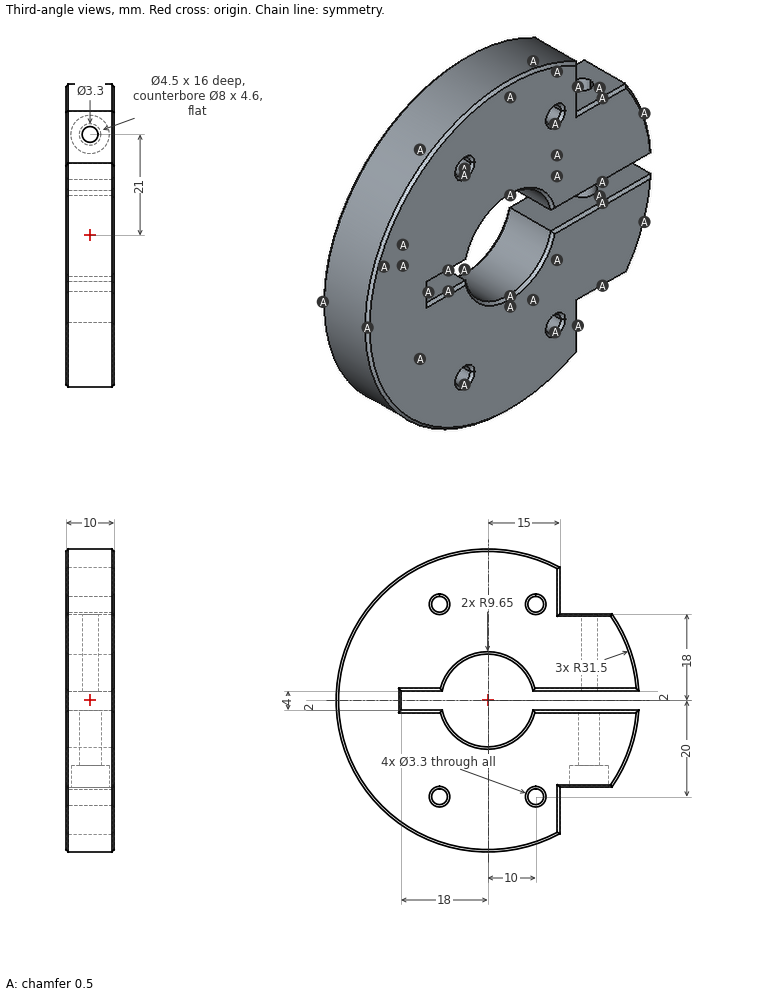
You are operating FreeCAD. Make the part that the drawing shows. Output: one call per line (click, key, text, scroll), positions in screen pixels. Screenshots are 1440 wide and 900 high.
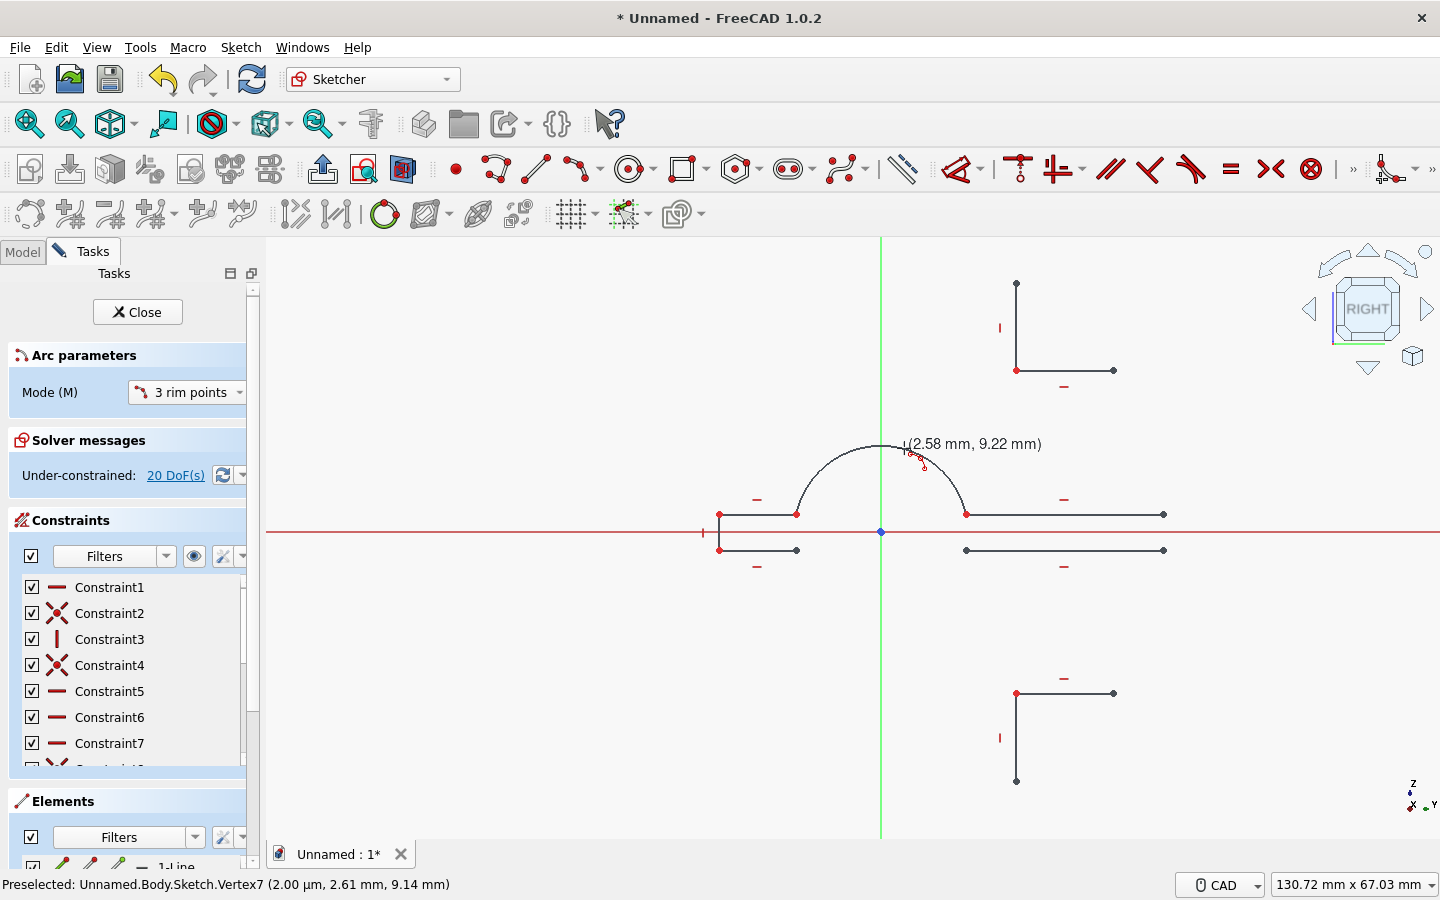
click(1163, 515)
click(1113, 371)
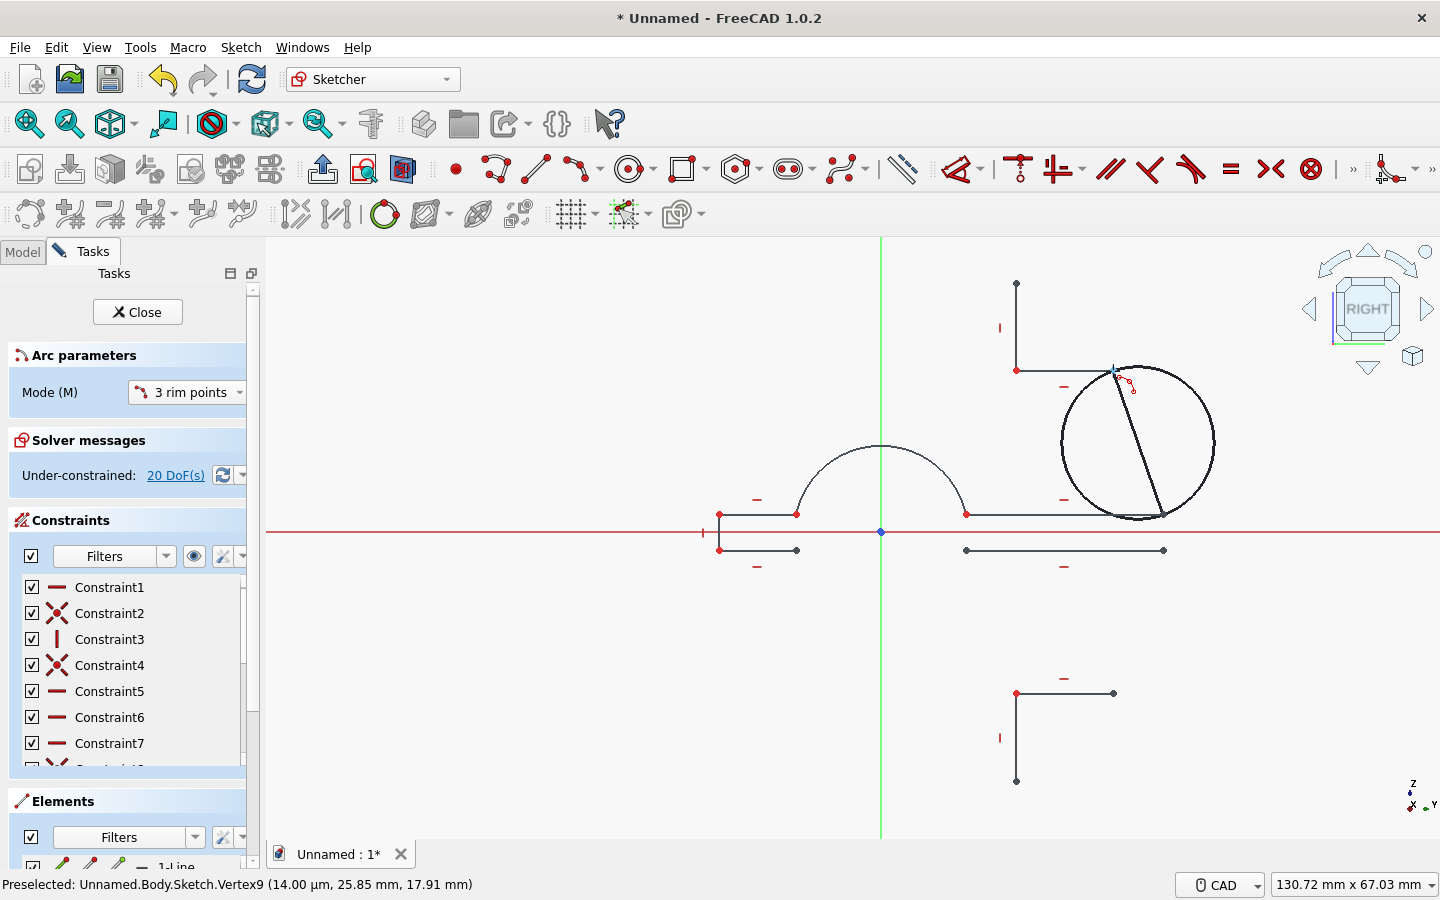
scroll(1148, 439, up, 3)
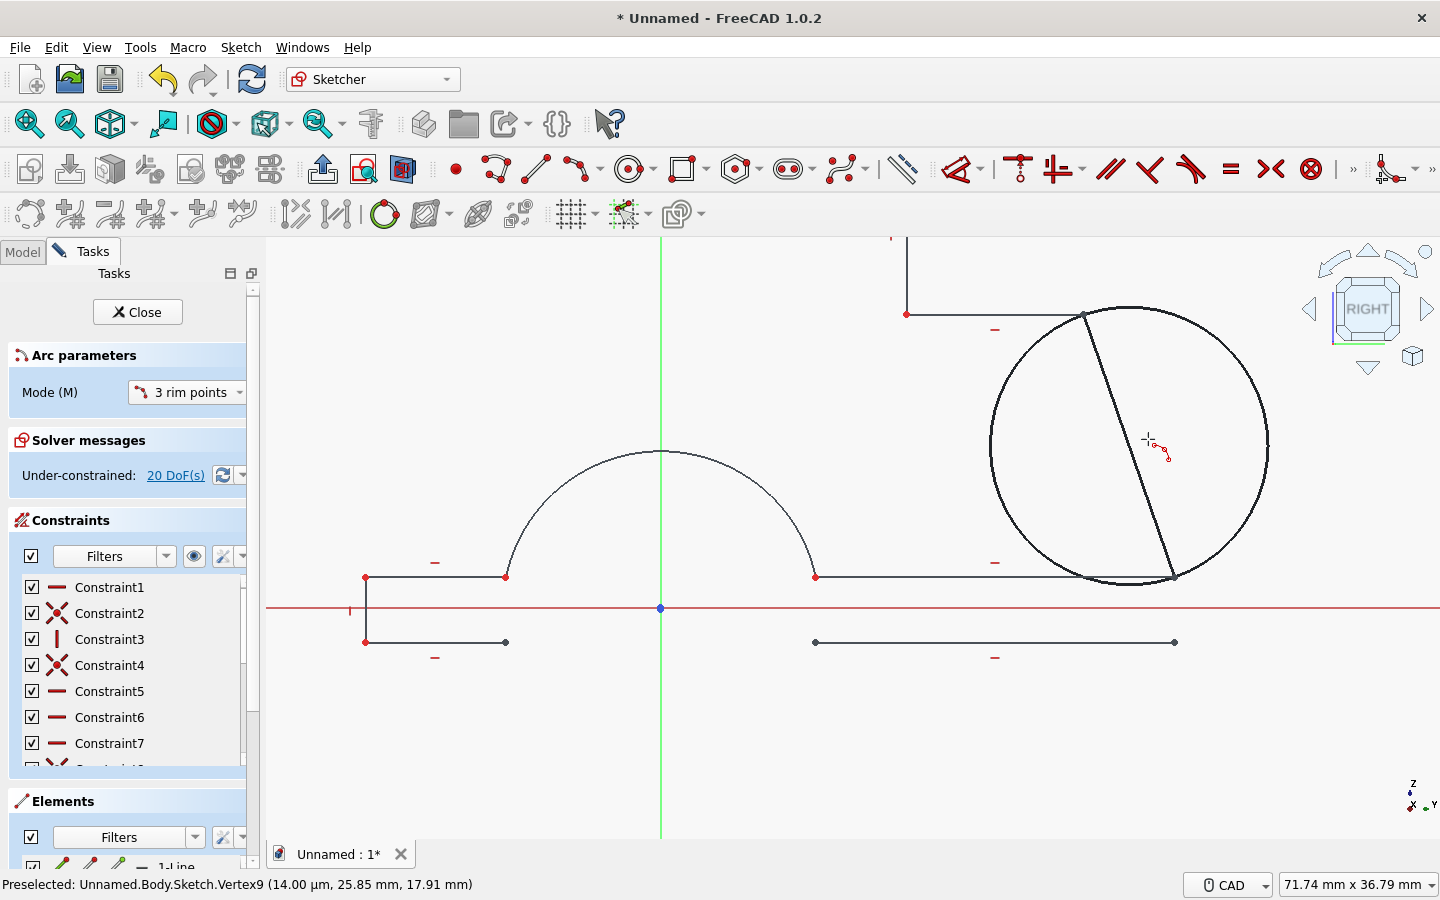
click(1147, 438)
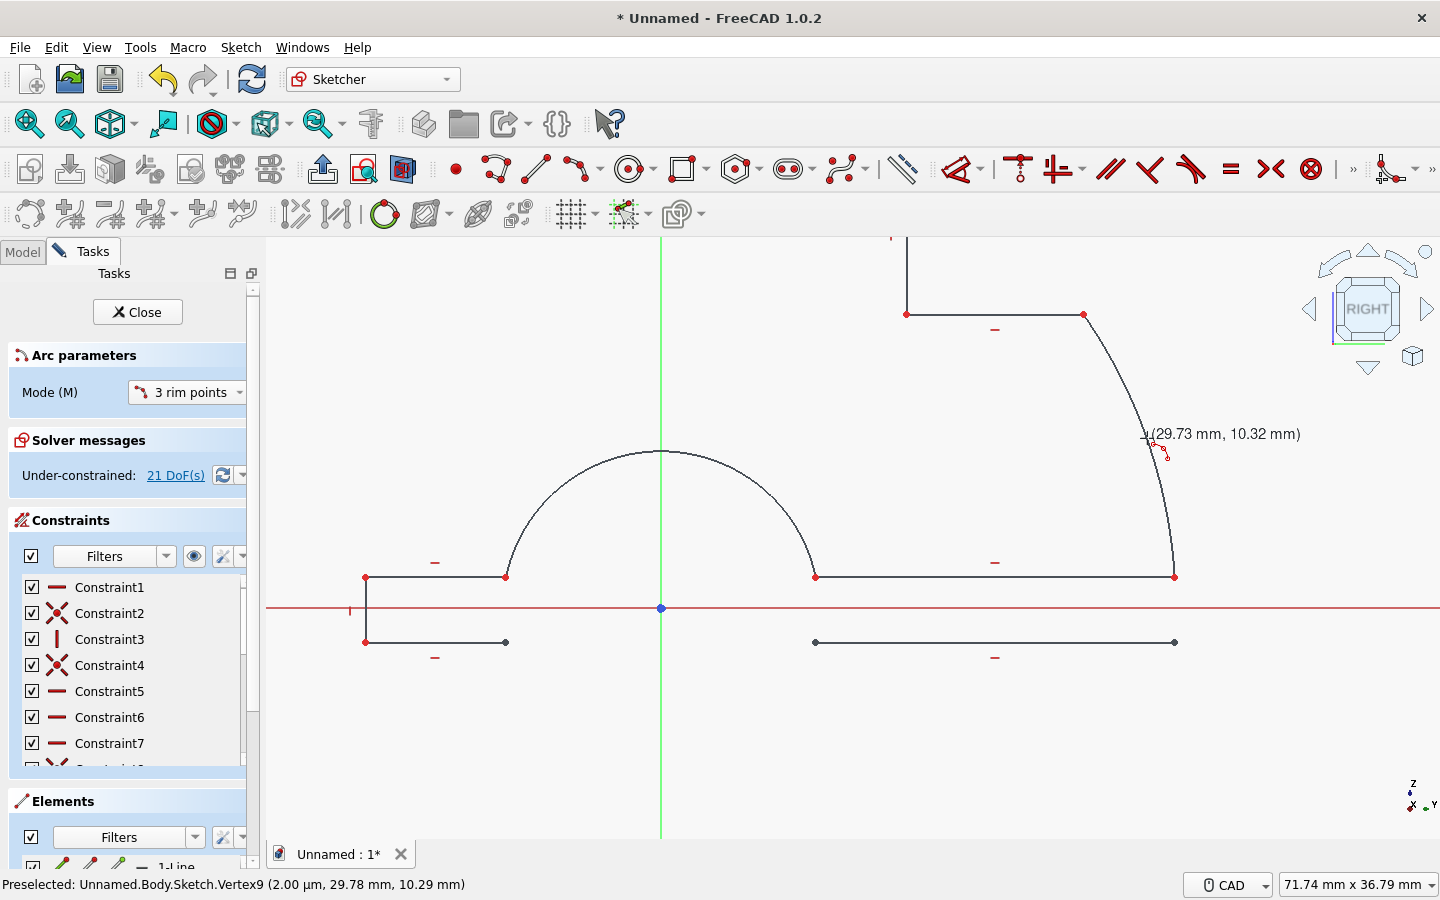
scroll(886, 481, down, 4)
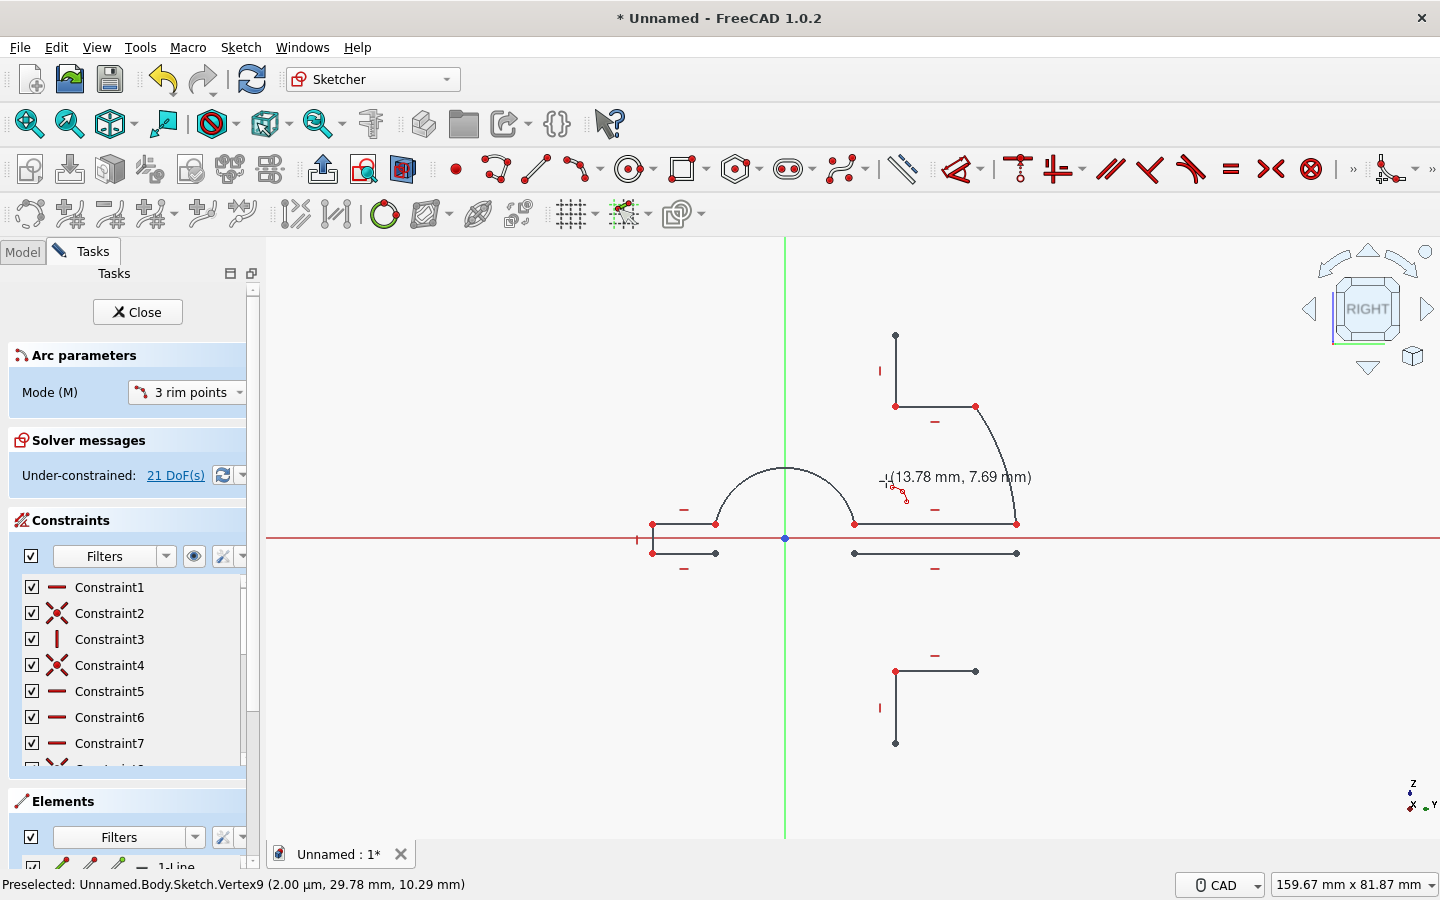
click(896, 335)
click(896, 743)
click(573, 445)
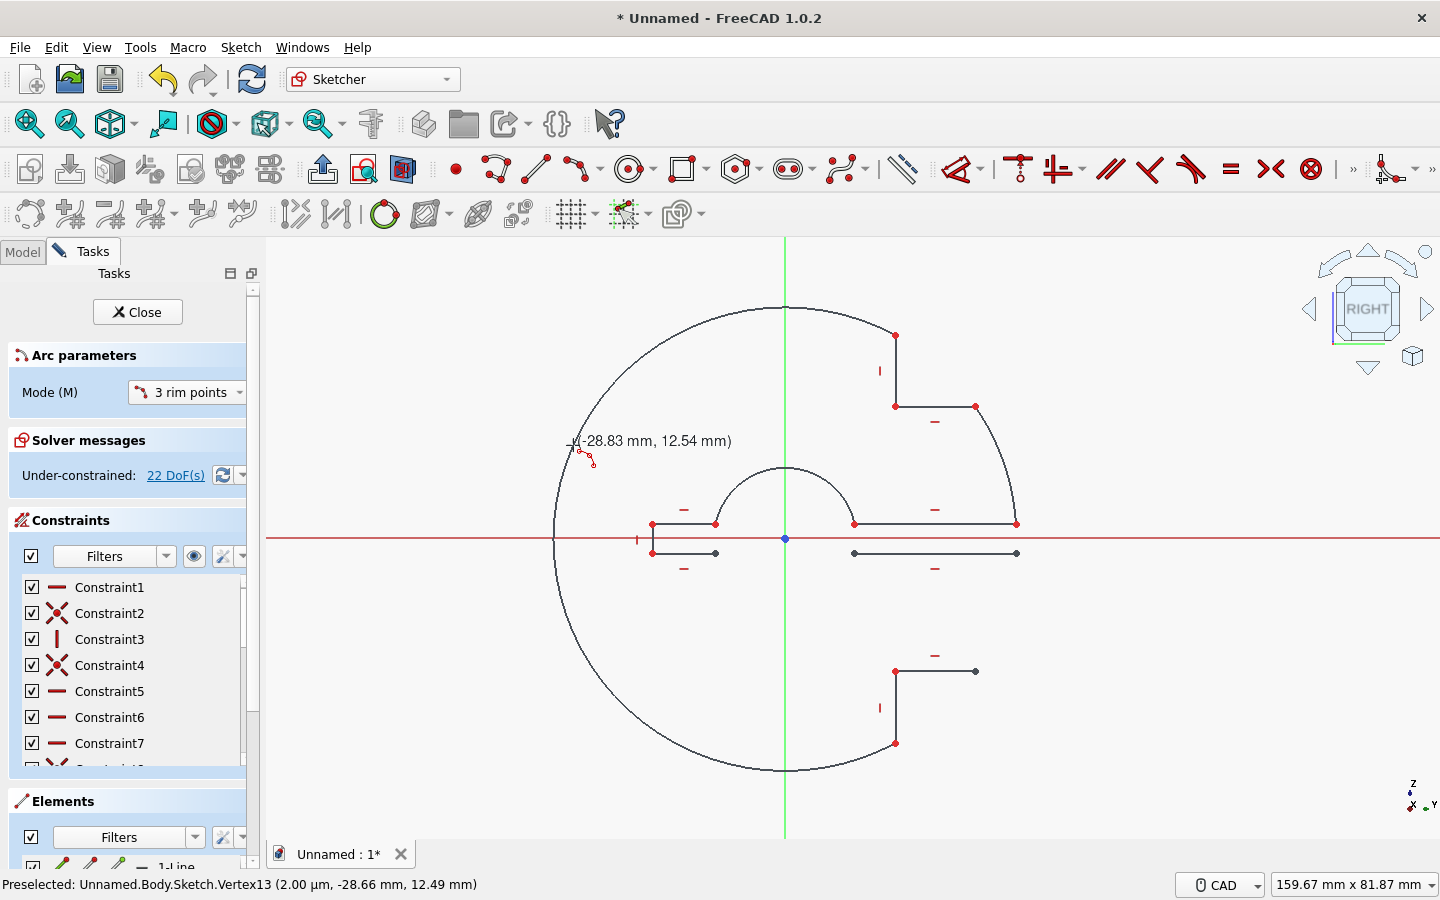
click(975, 671)
click(1016, 554)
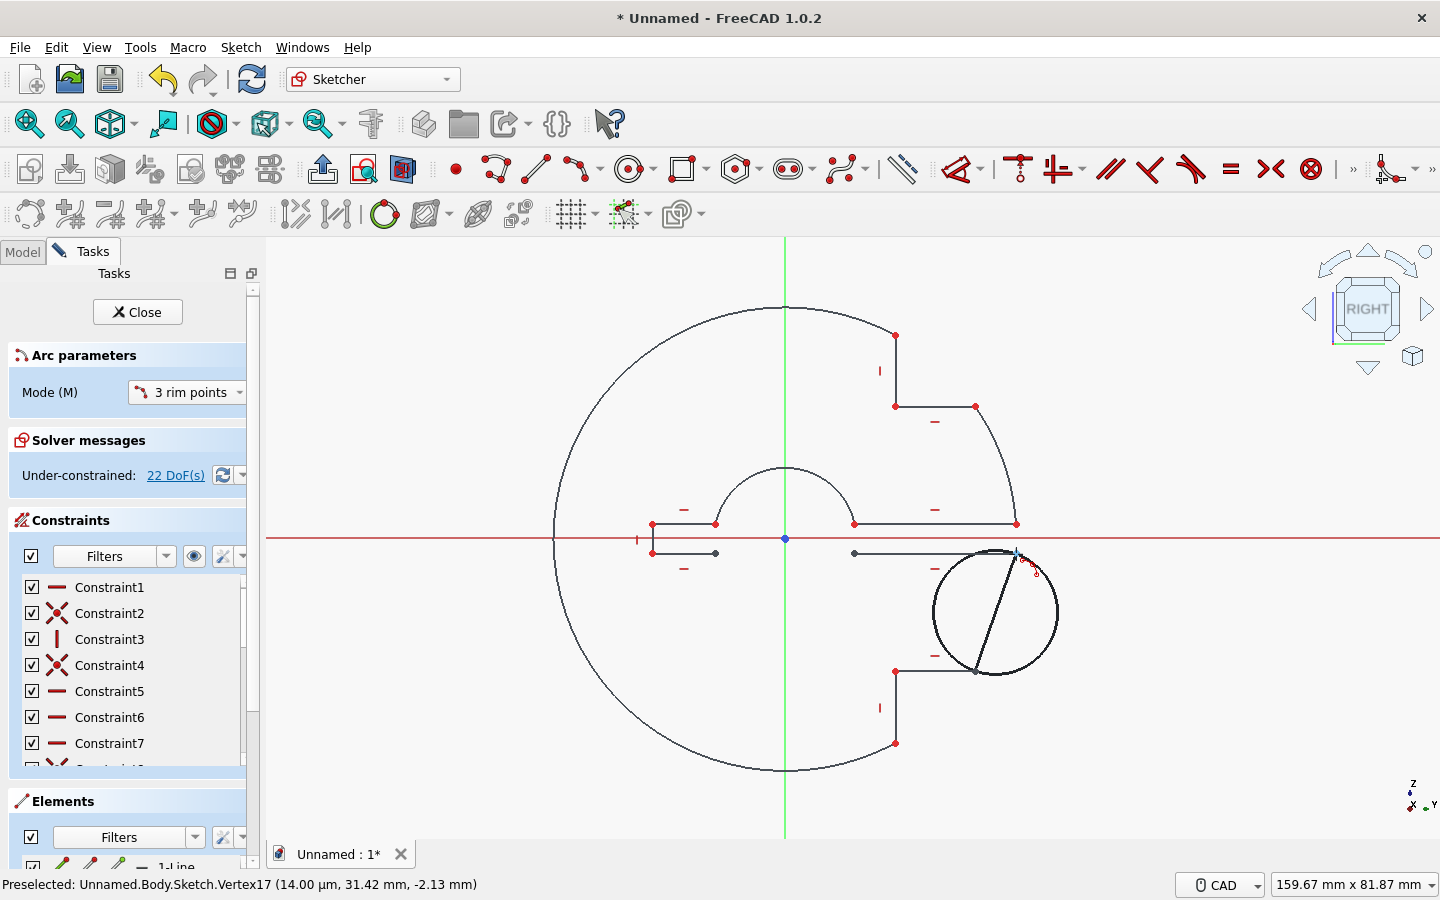
scroll(1004, 615, up, 4)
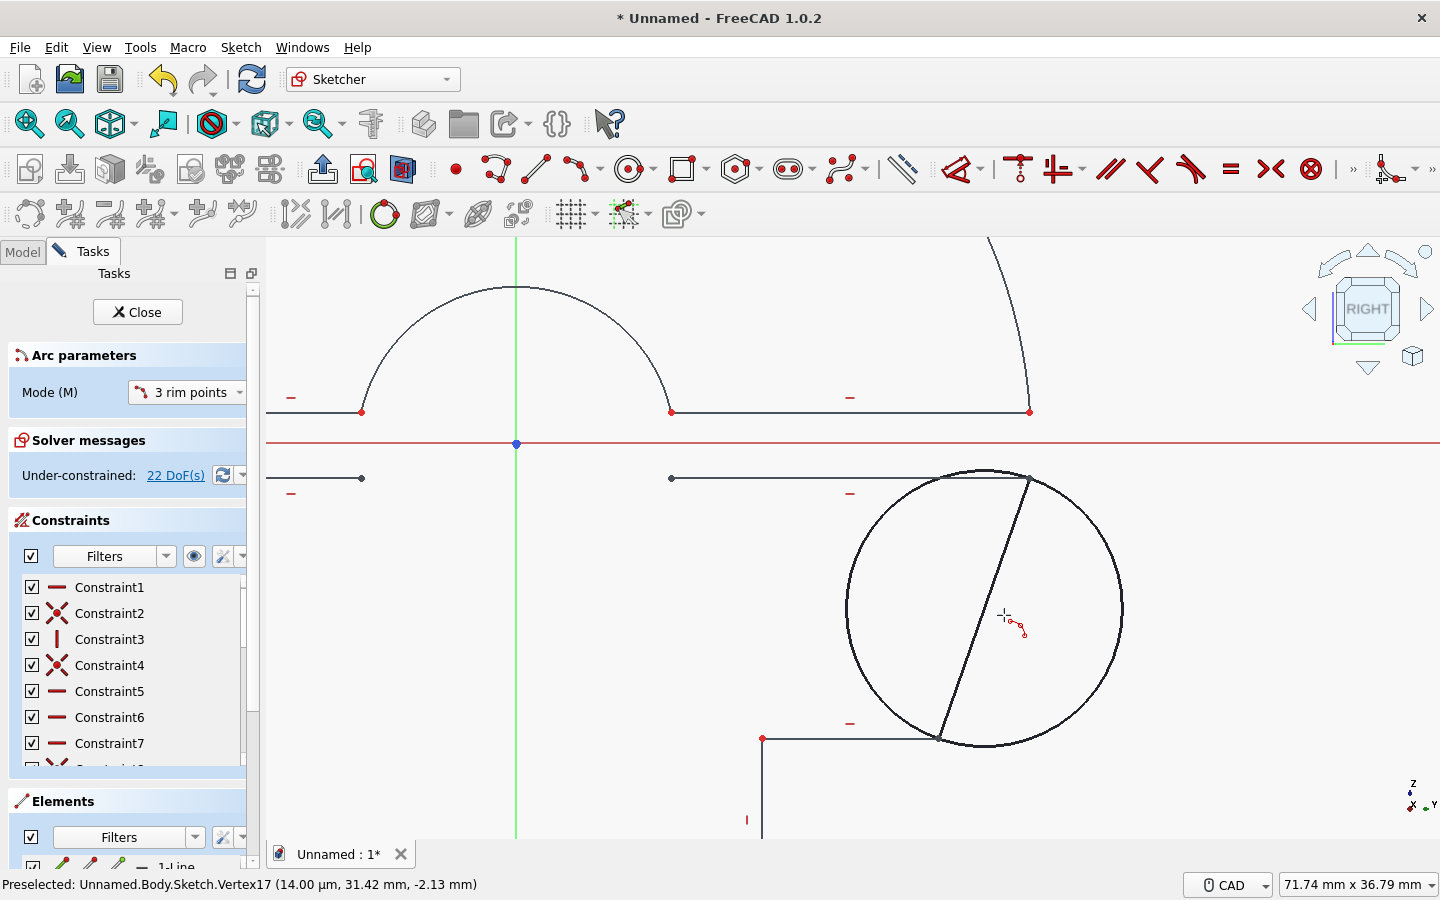
click(1002, 613)